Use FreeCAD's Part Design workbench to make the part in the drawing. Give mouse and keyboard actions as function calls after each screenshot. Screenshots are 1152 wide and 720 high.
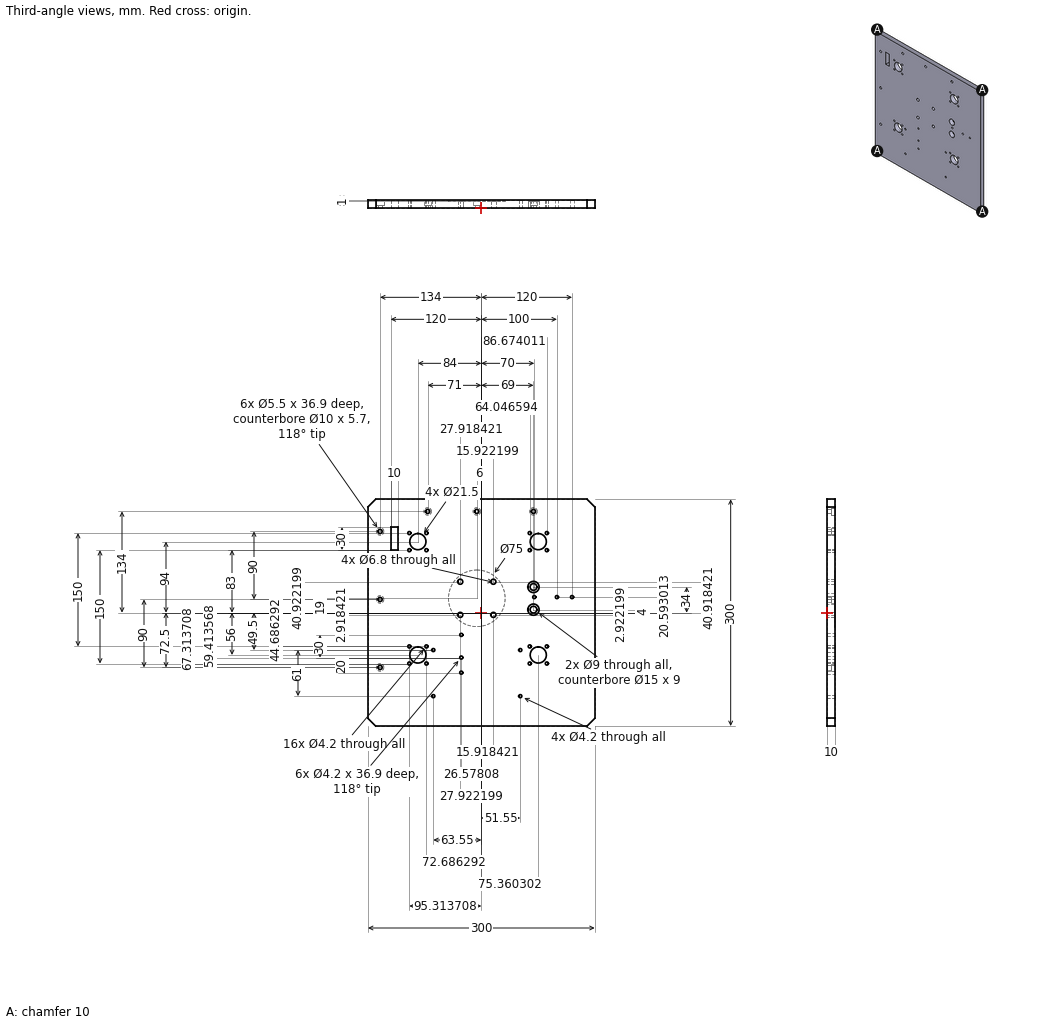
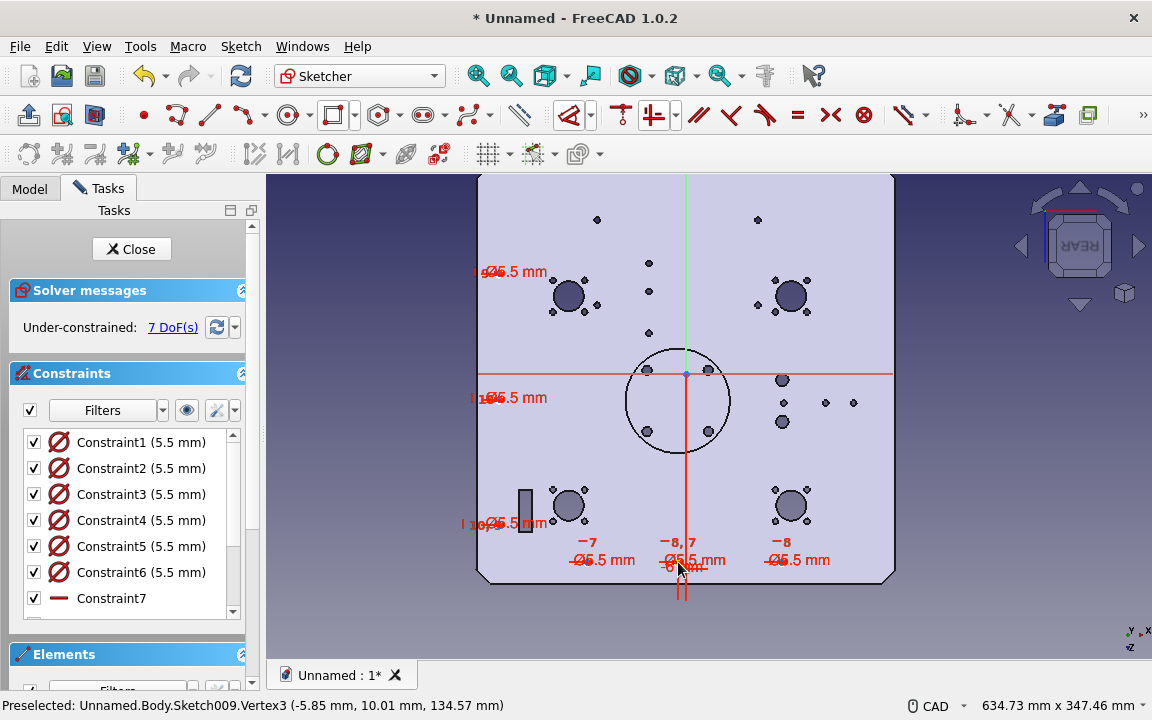
click(587, 562)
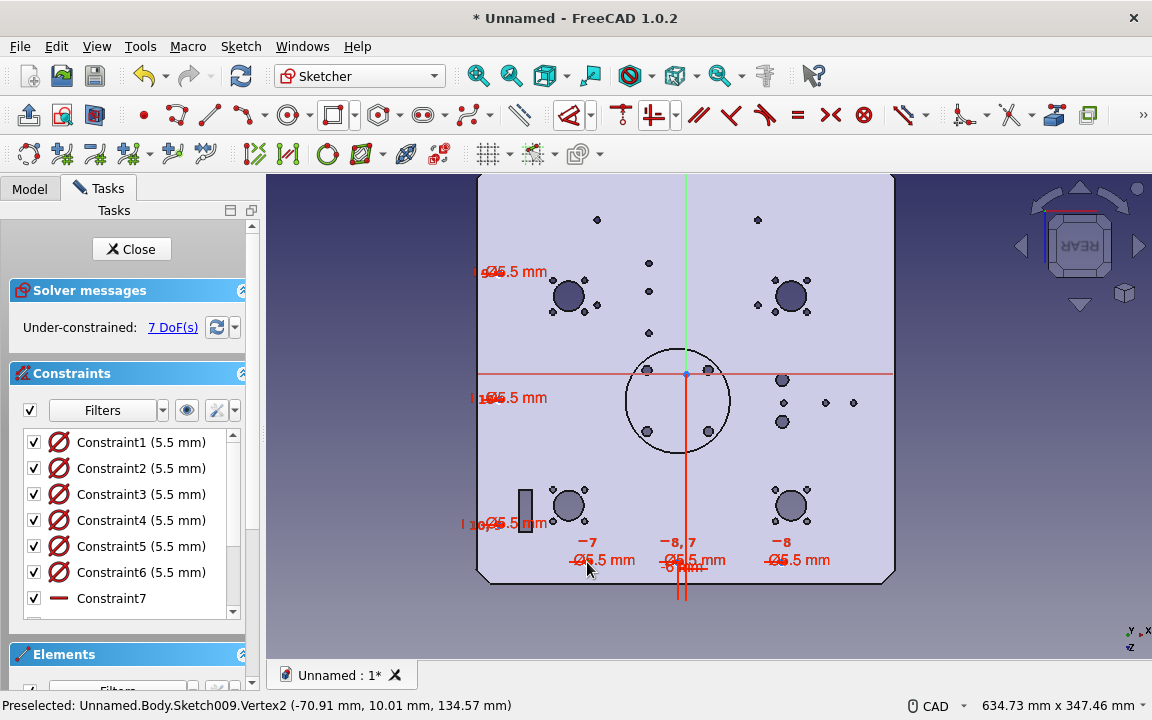
key(l)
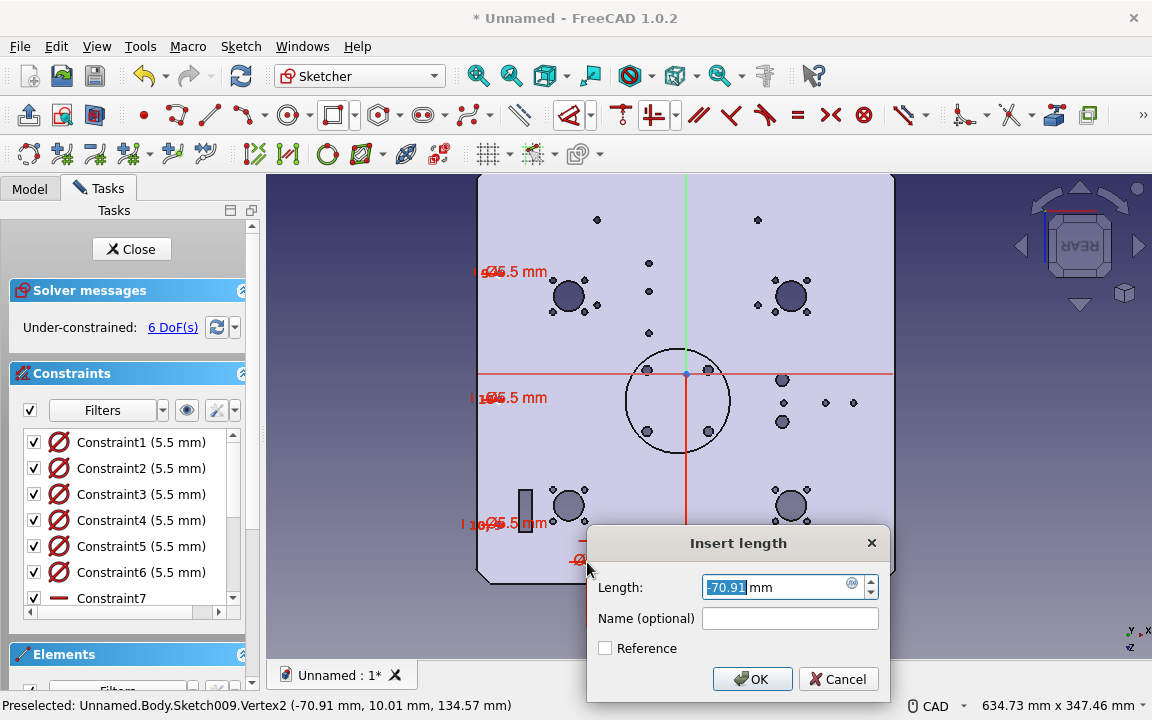
text(-71)
key(Return)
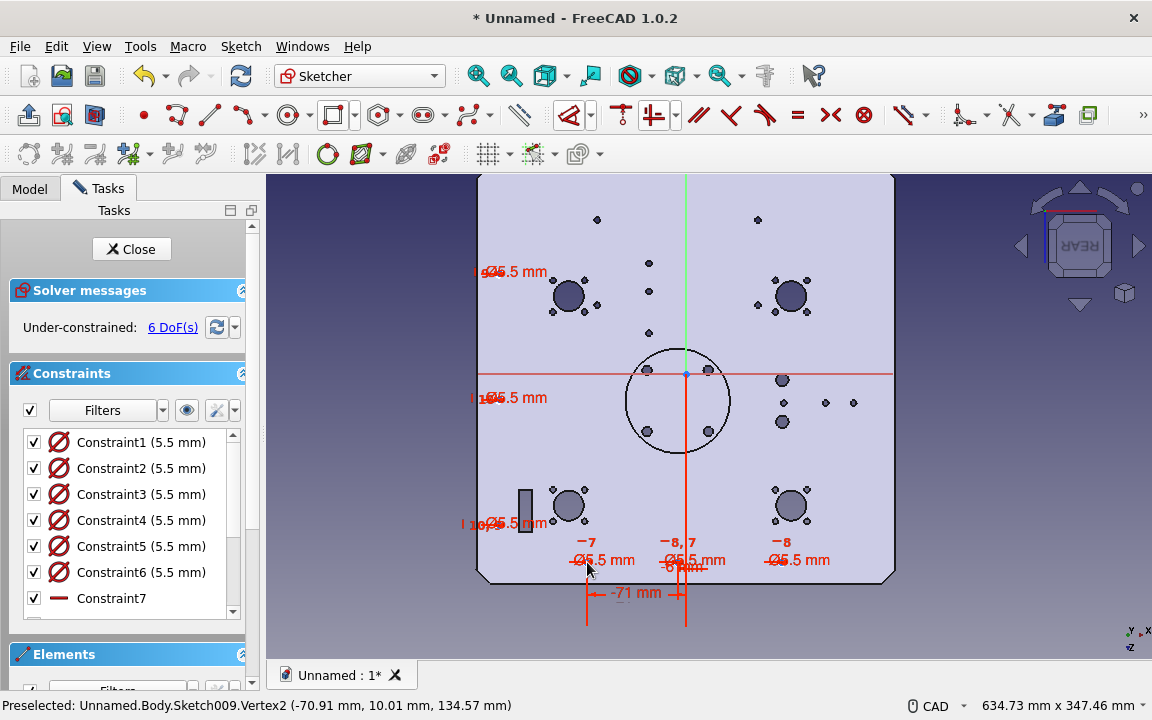
click(782, 562)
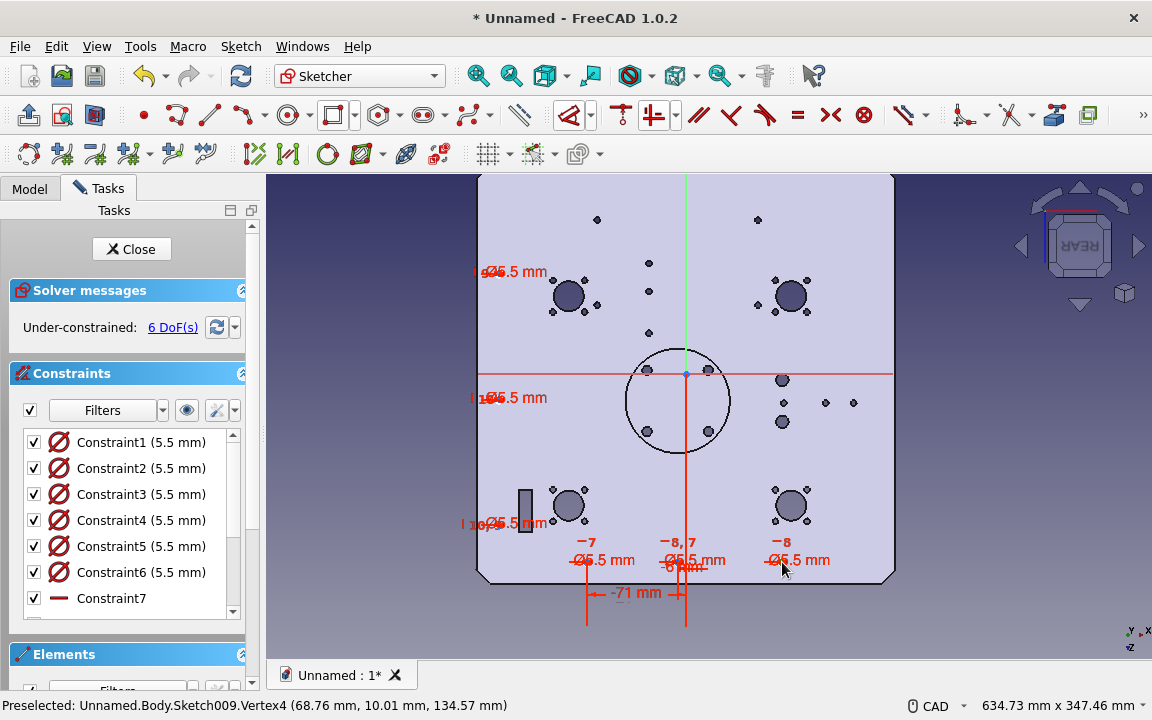
key(l)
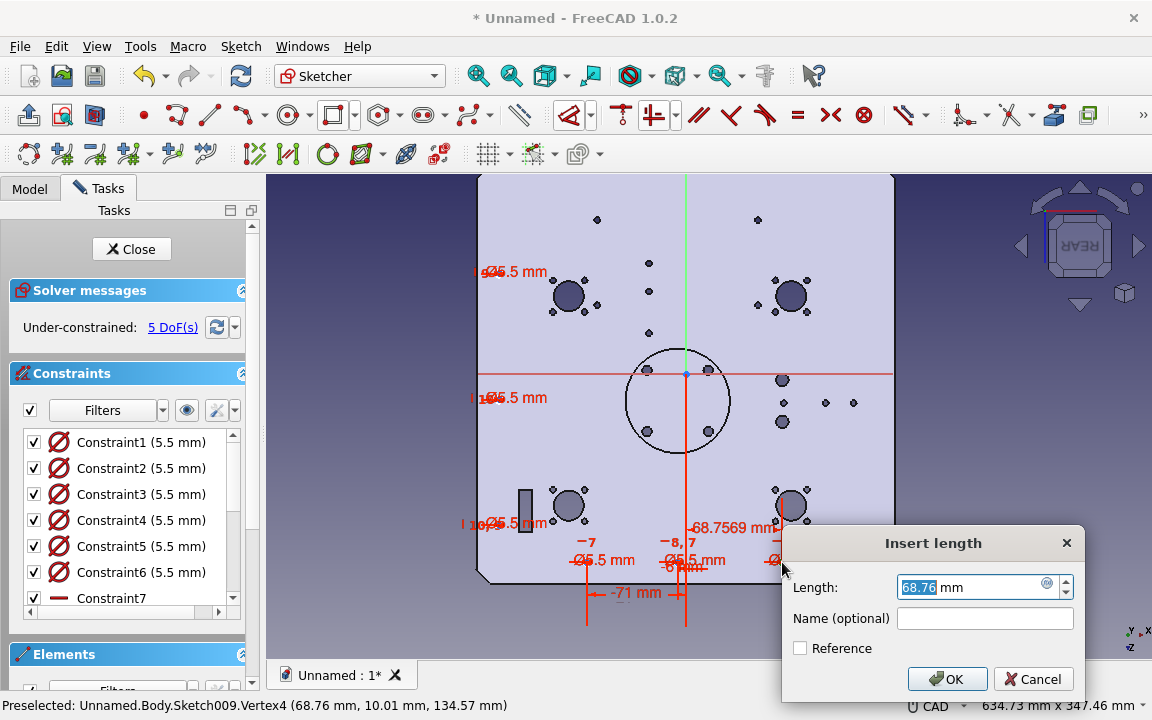
text(69)
key(Return)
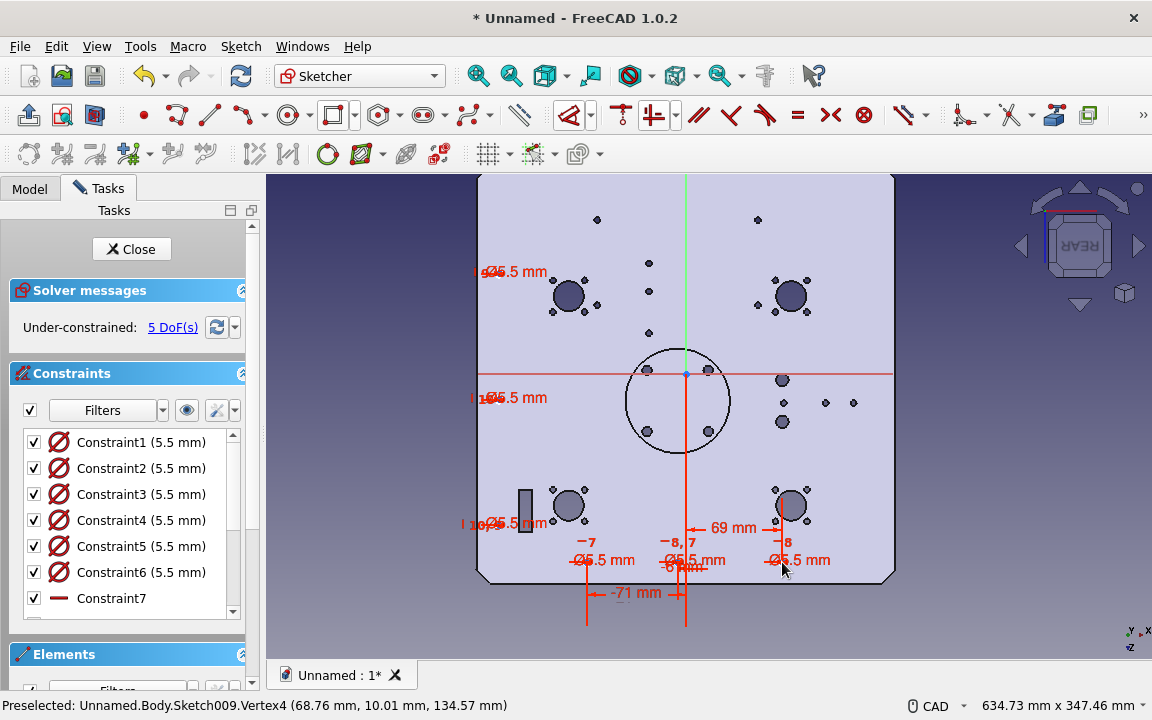
click(499, 525)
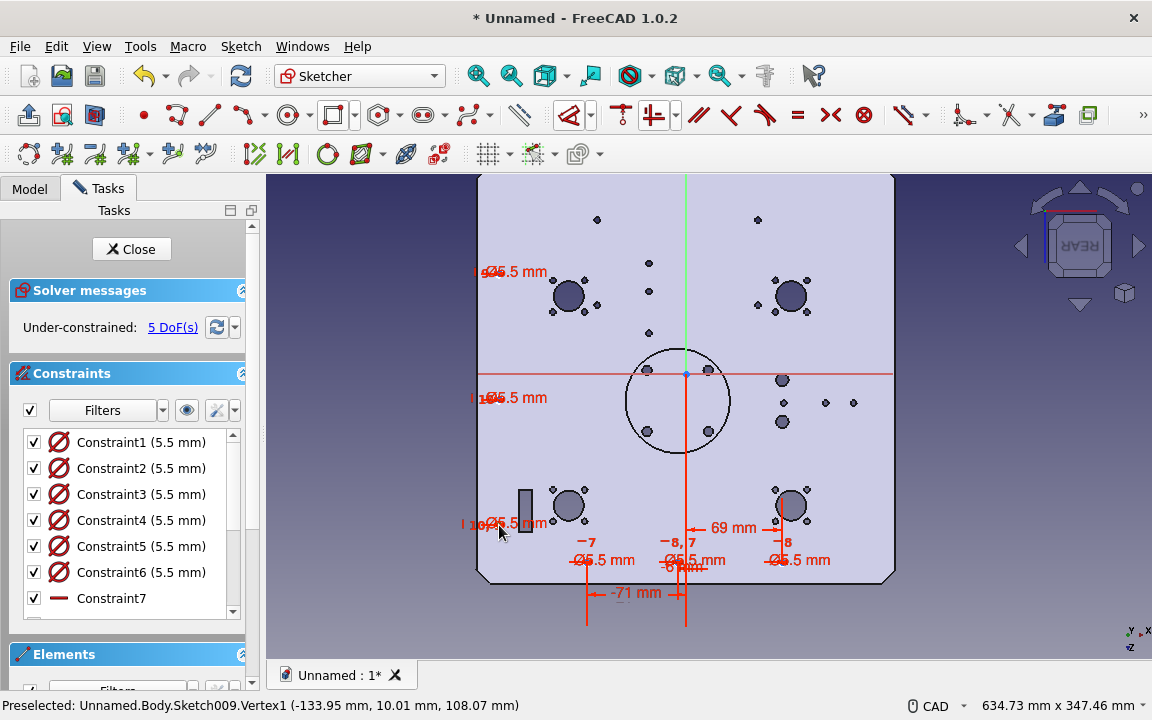
click(590, 116)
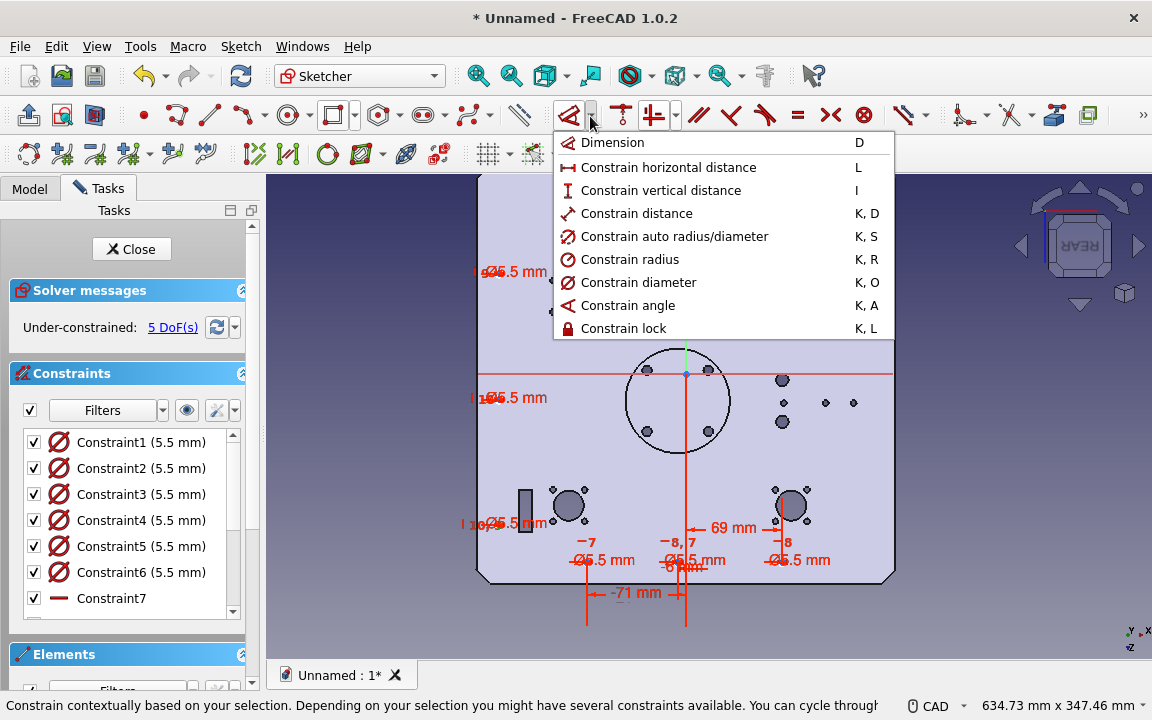
click(724, 168)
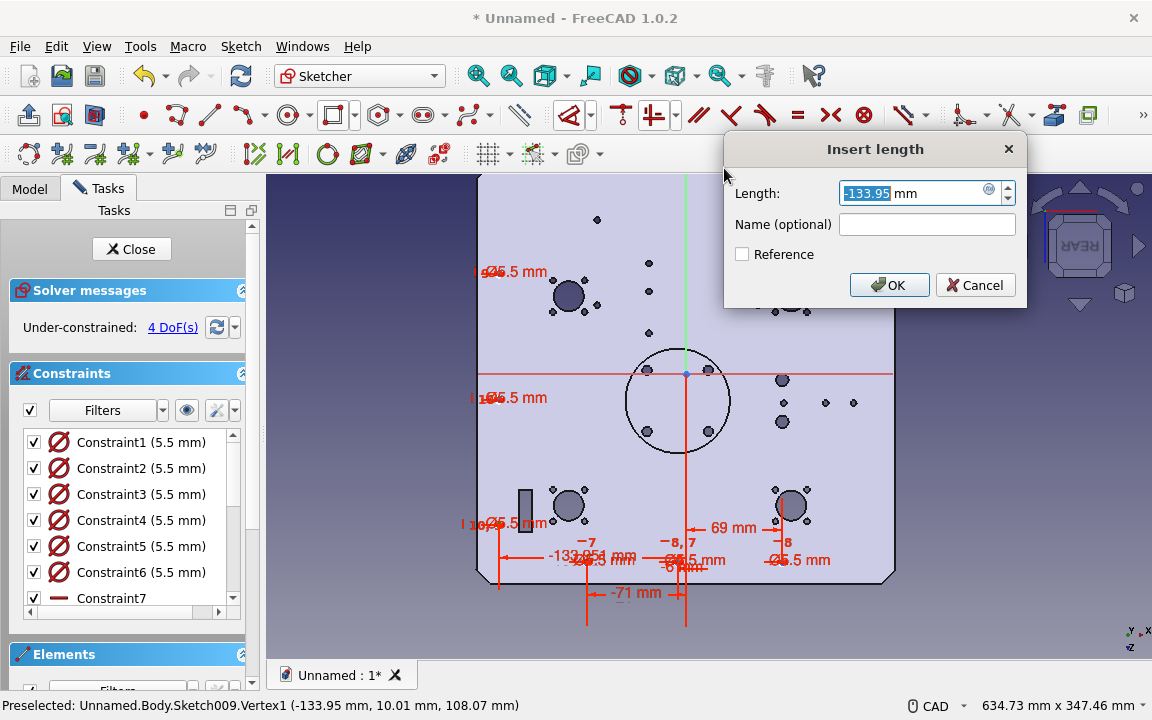
text(-134)
key(Return)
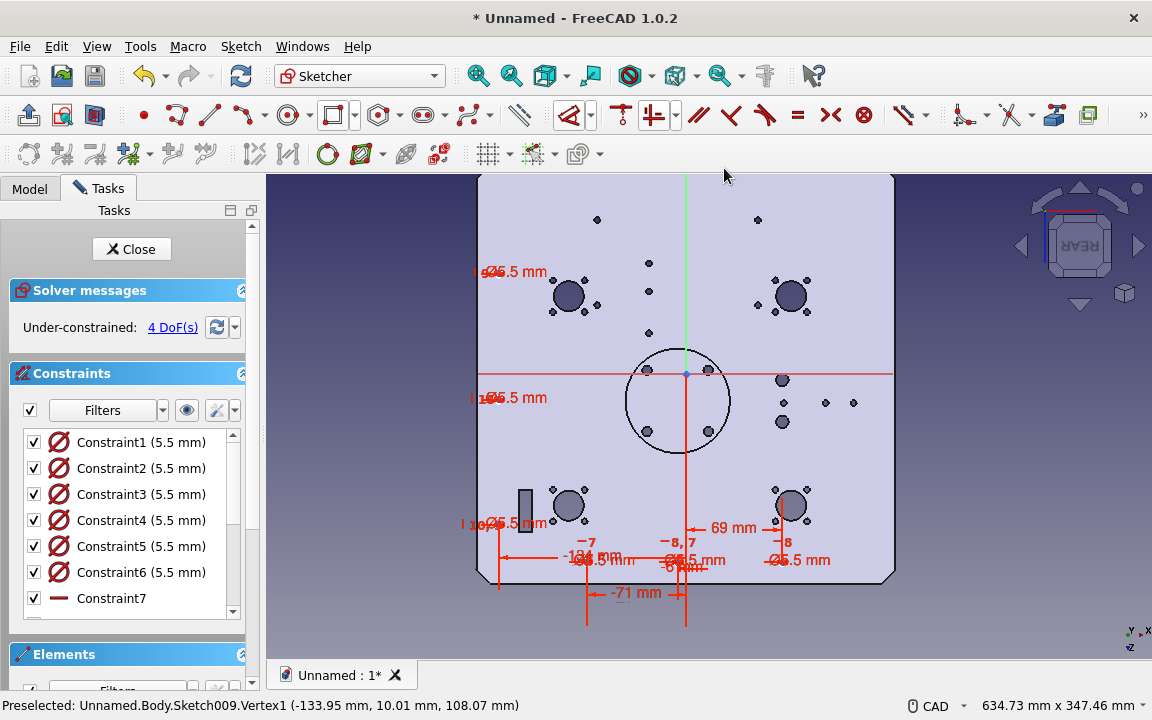
click(587, 562)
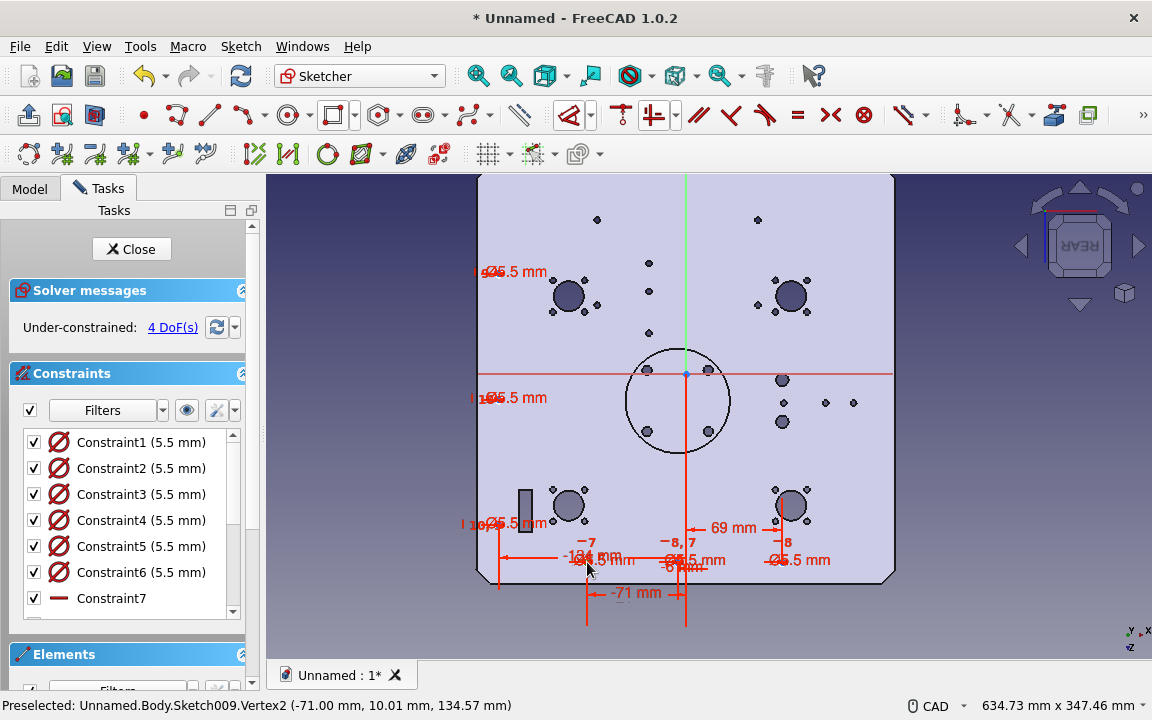
click(590, 116)